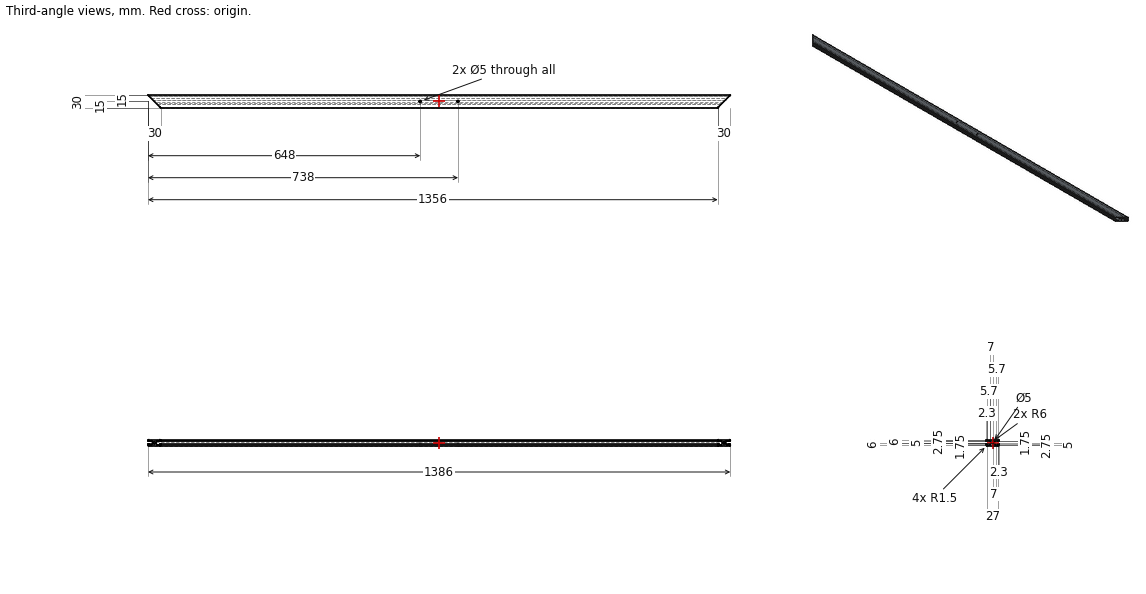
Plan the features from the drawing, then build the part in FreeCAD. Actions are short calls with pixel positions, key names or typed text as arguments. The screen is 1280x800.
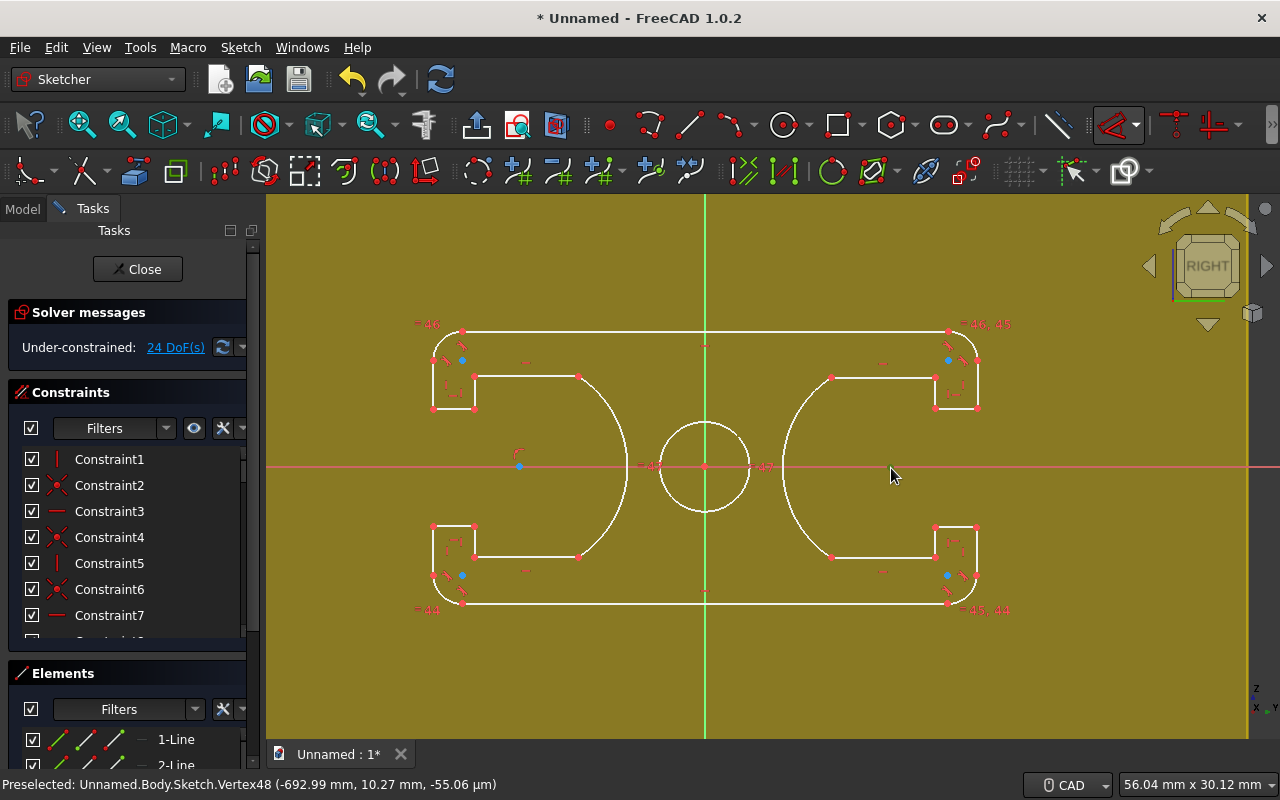
click(353, 467)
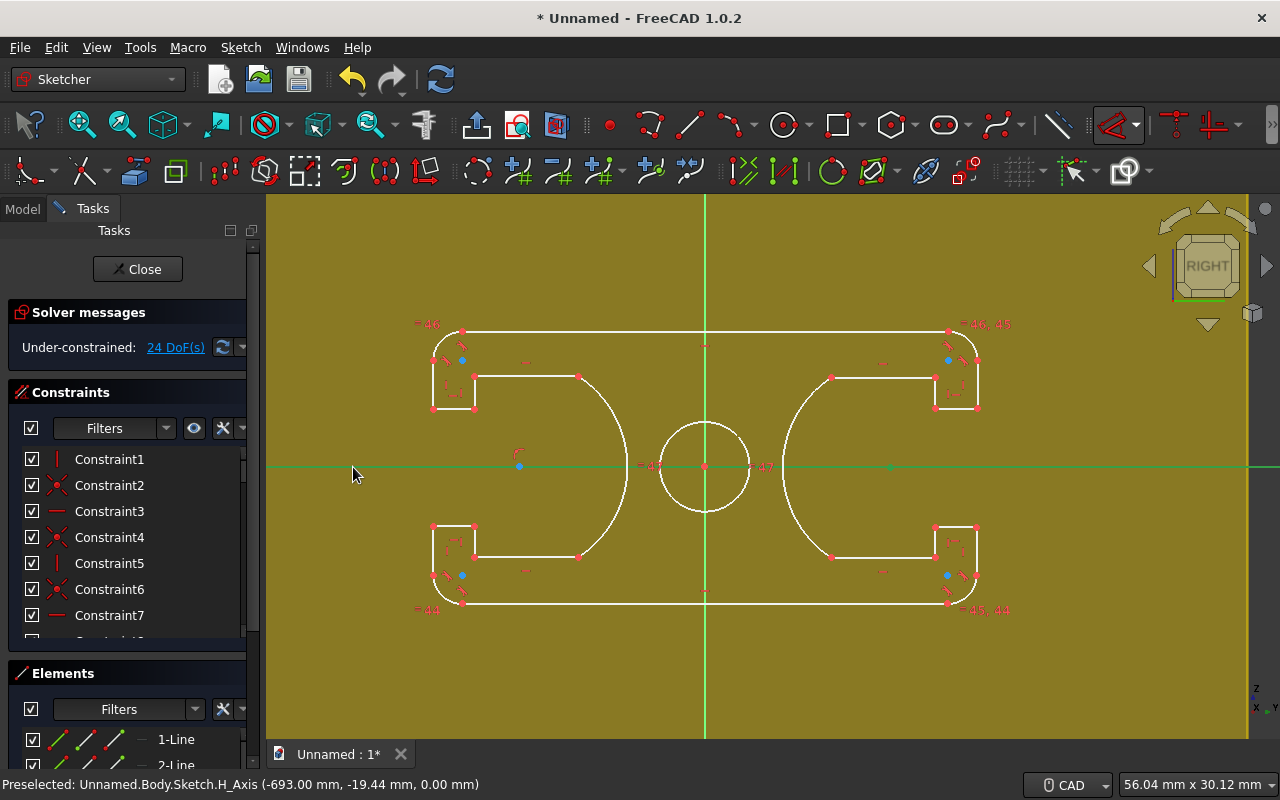
click(1174, 126)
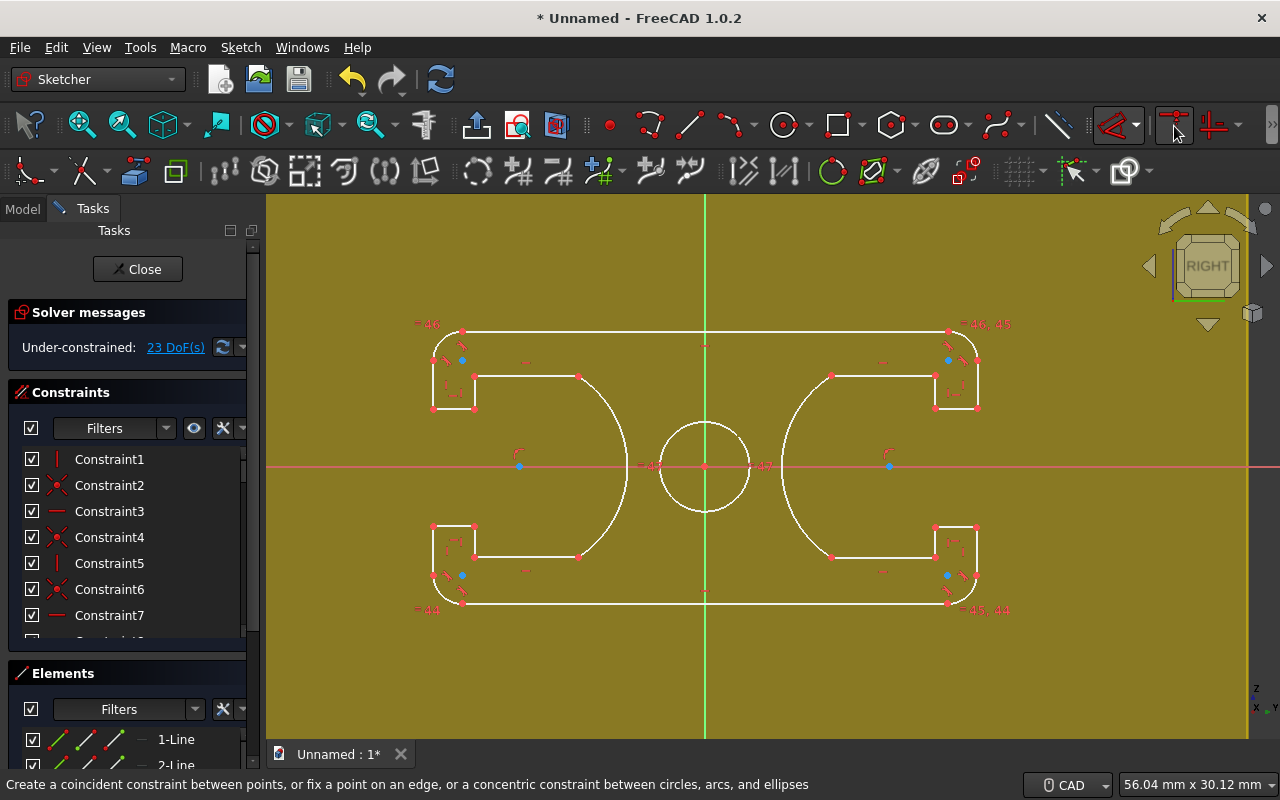
click(619, 508)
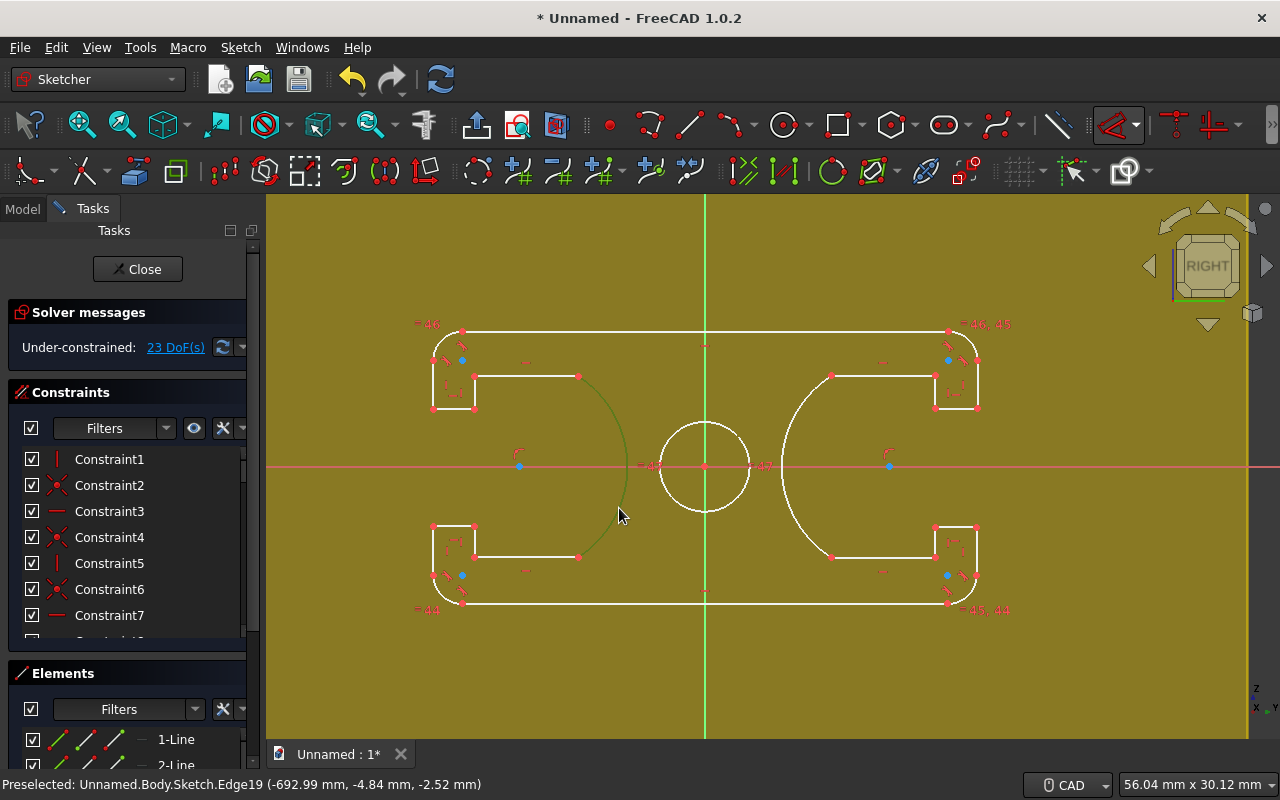
key(k)
key(r)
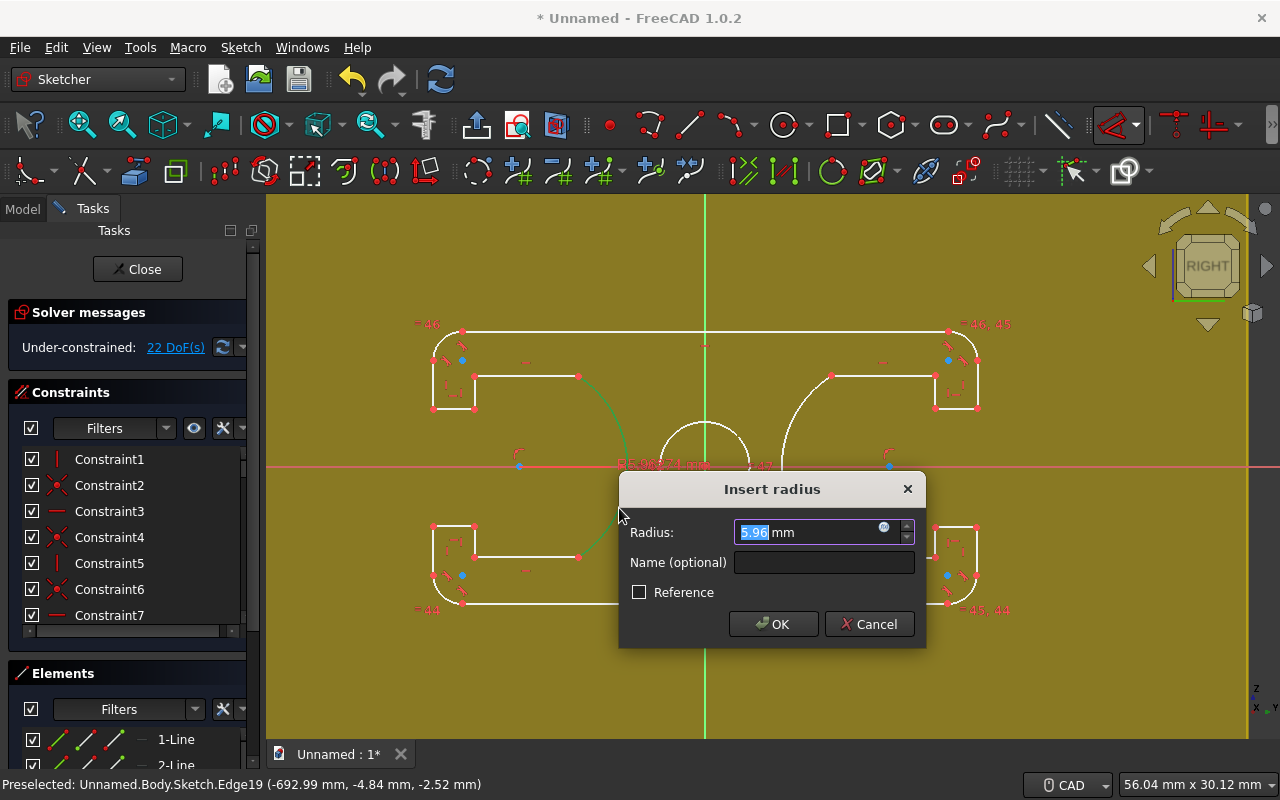
text(6)
key(Return)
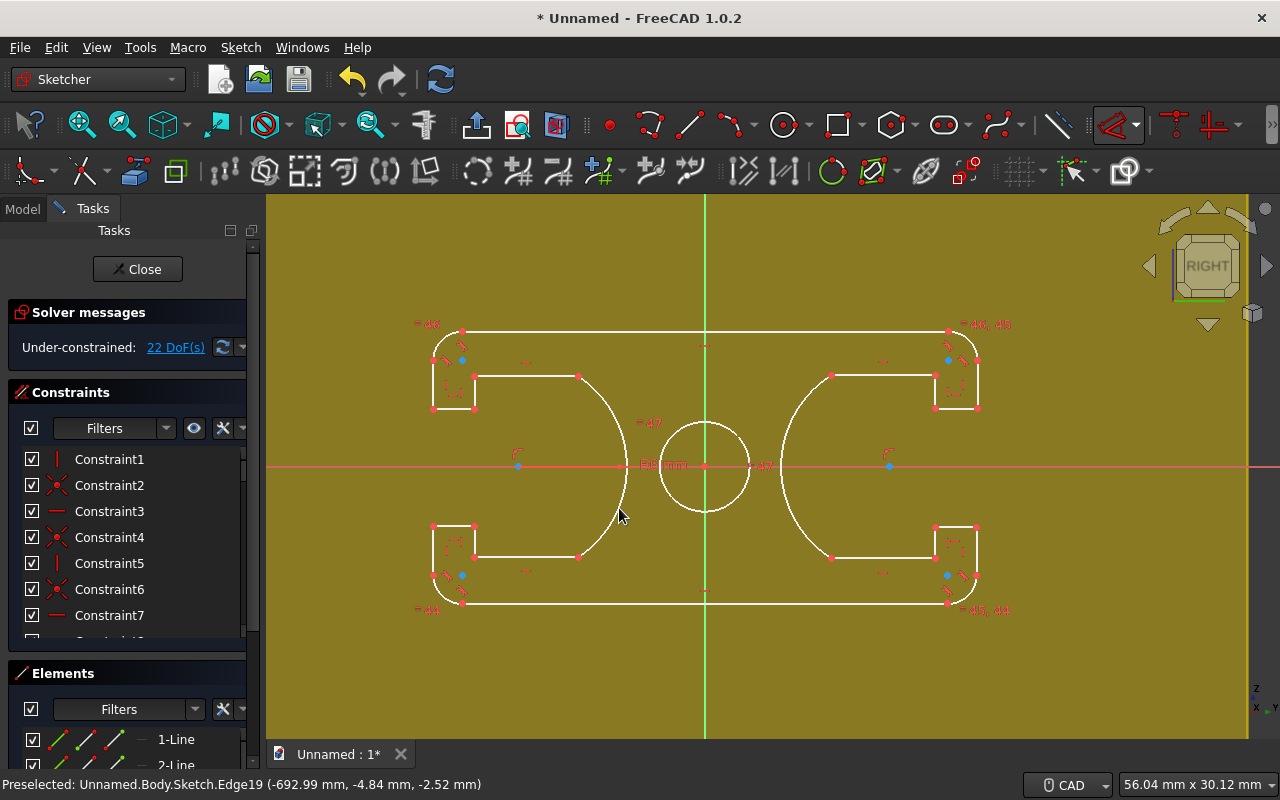
scroll(437, 588, up, 2)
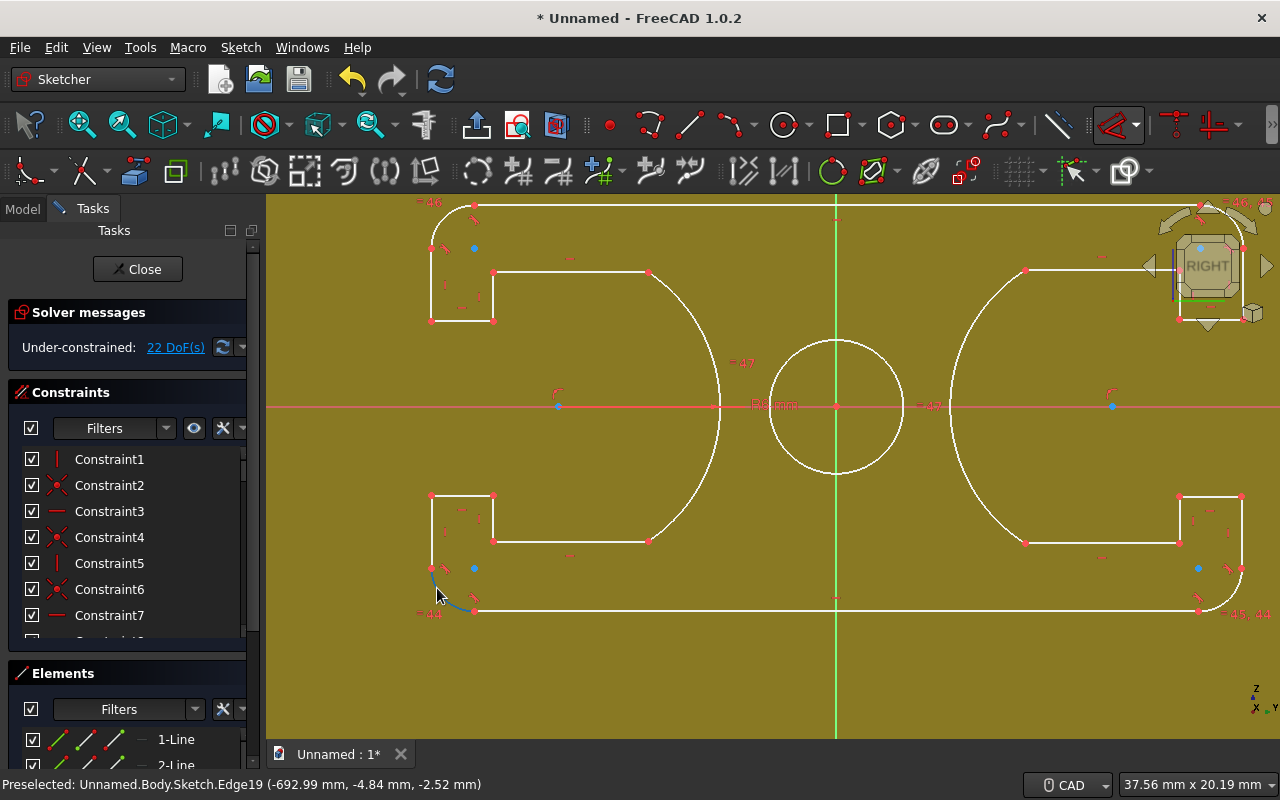
click(436, 588)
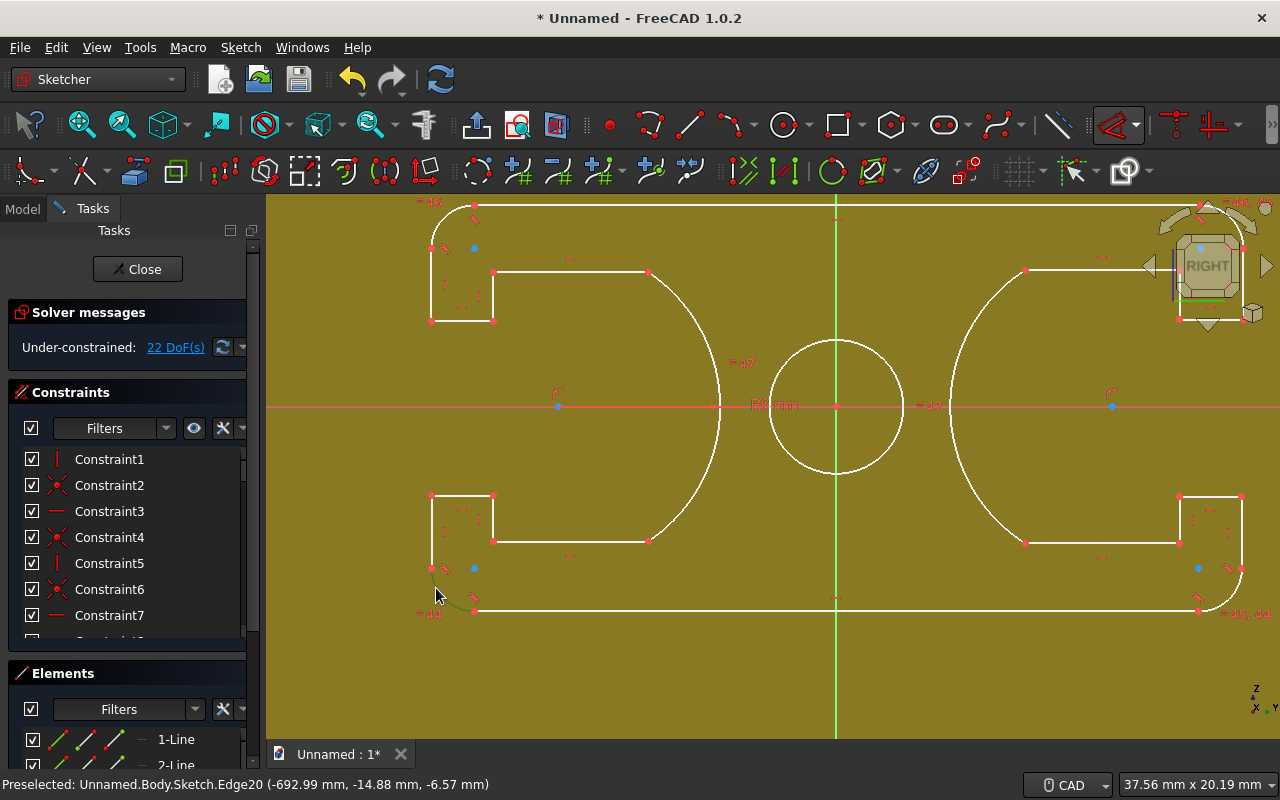
click(1138, 126)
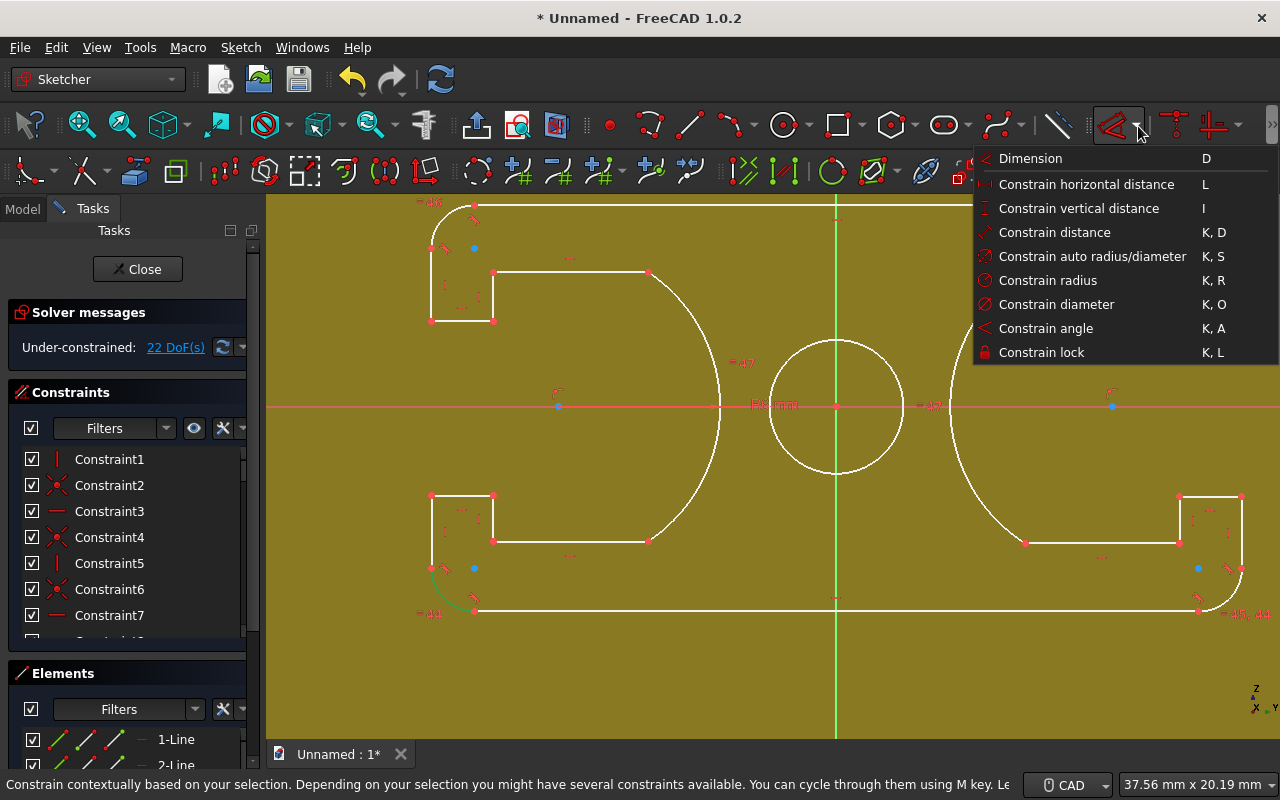
click(1126, 280)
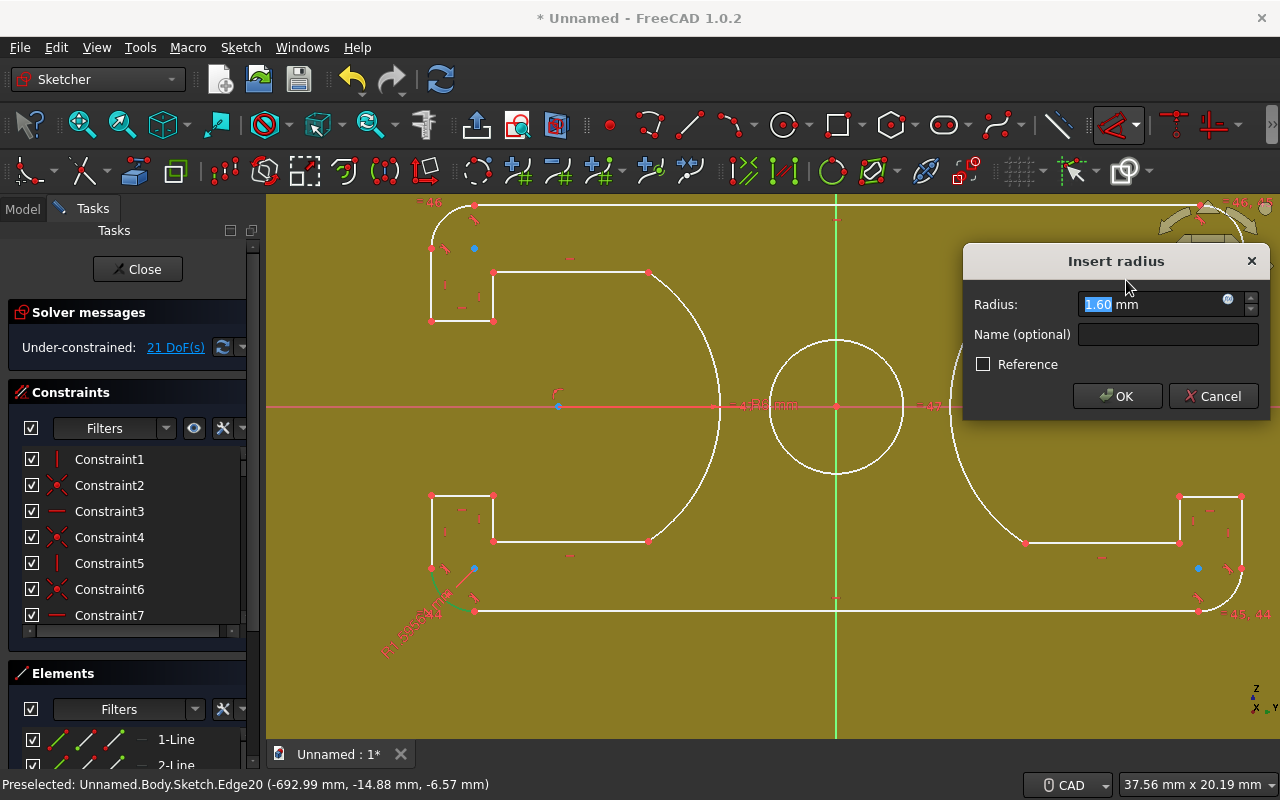
text(1.5)
key(Return)